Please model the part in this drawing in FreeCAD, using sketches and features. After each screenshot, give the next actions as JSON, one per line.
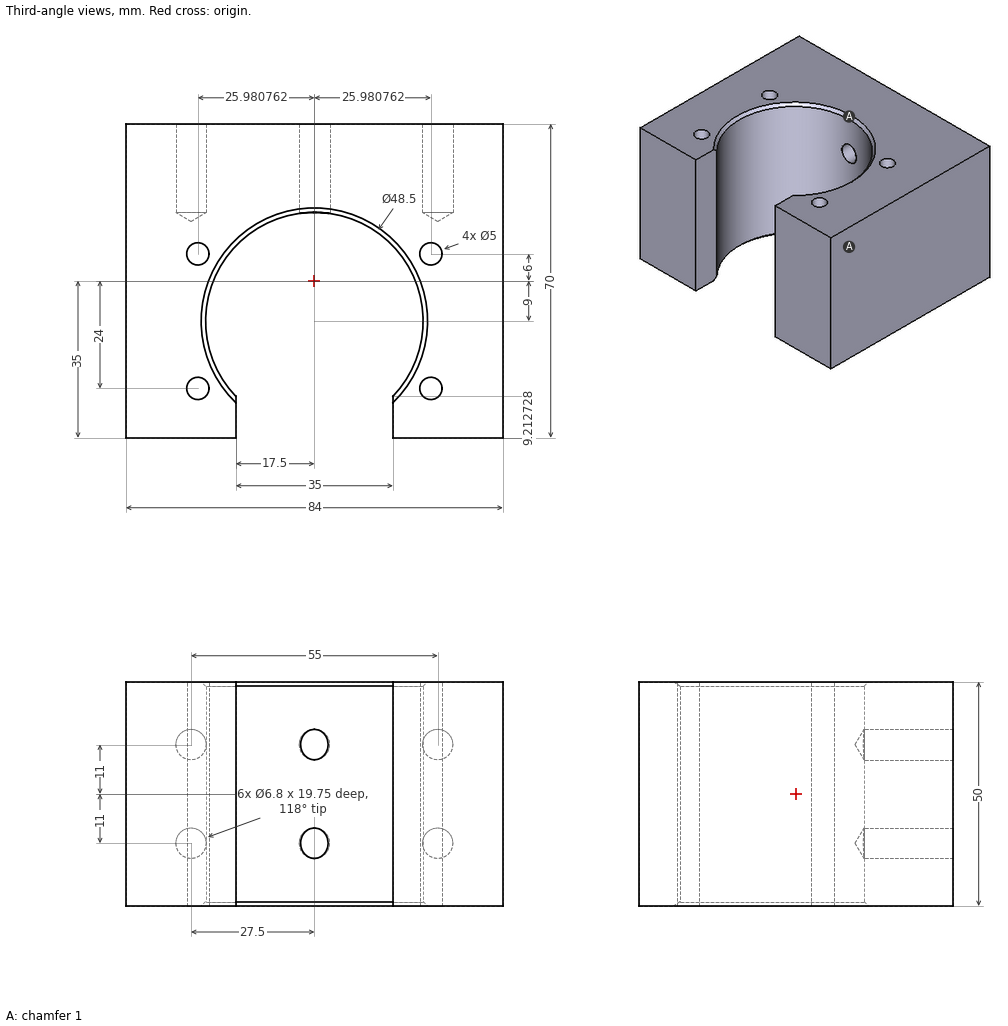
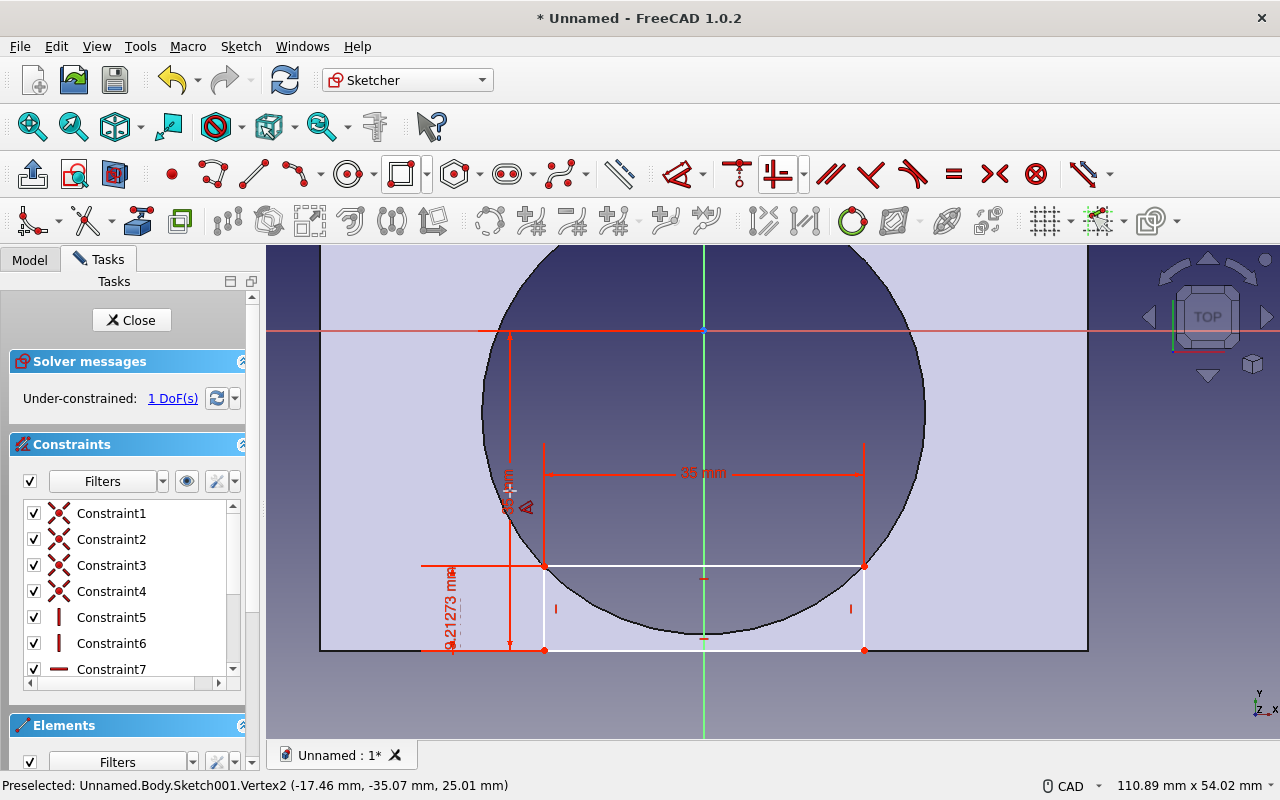
{"action": "left_click", "coordinate": [544, 566]}
{"action": "left_click", "coordinate": [624, 297]}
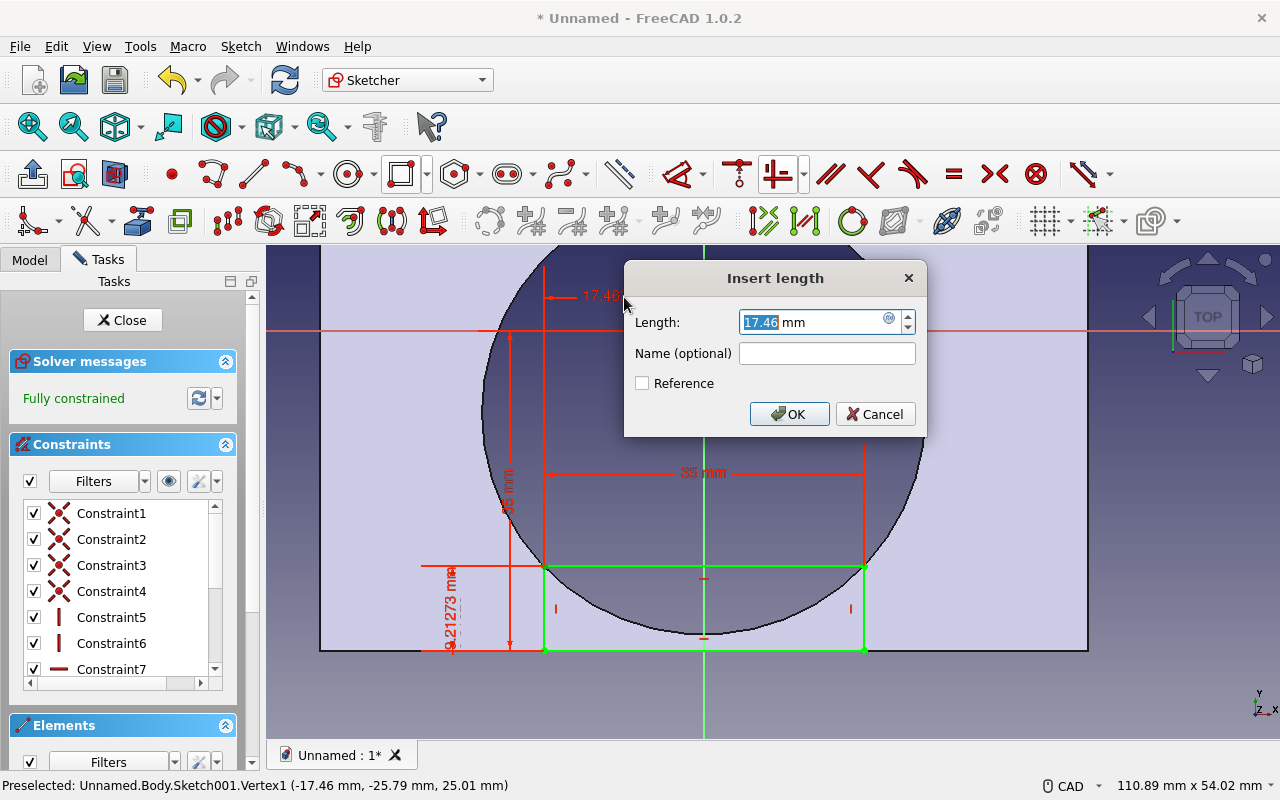
{"action": "type", "text": "17.5"}
{"action": "key", "text": "Return"}
{"action": "key", "text": "Escape"}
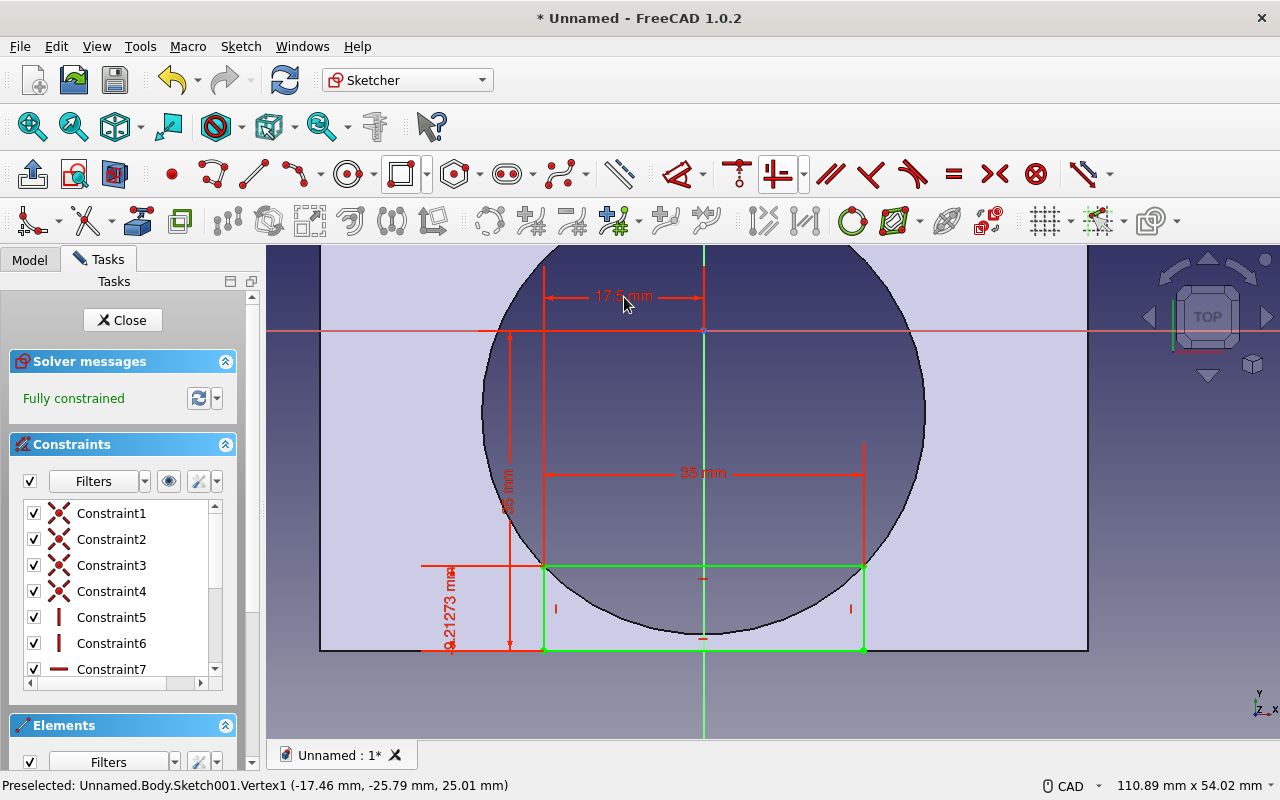
{"action": "left_click", "coordinate": [123, 320]}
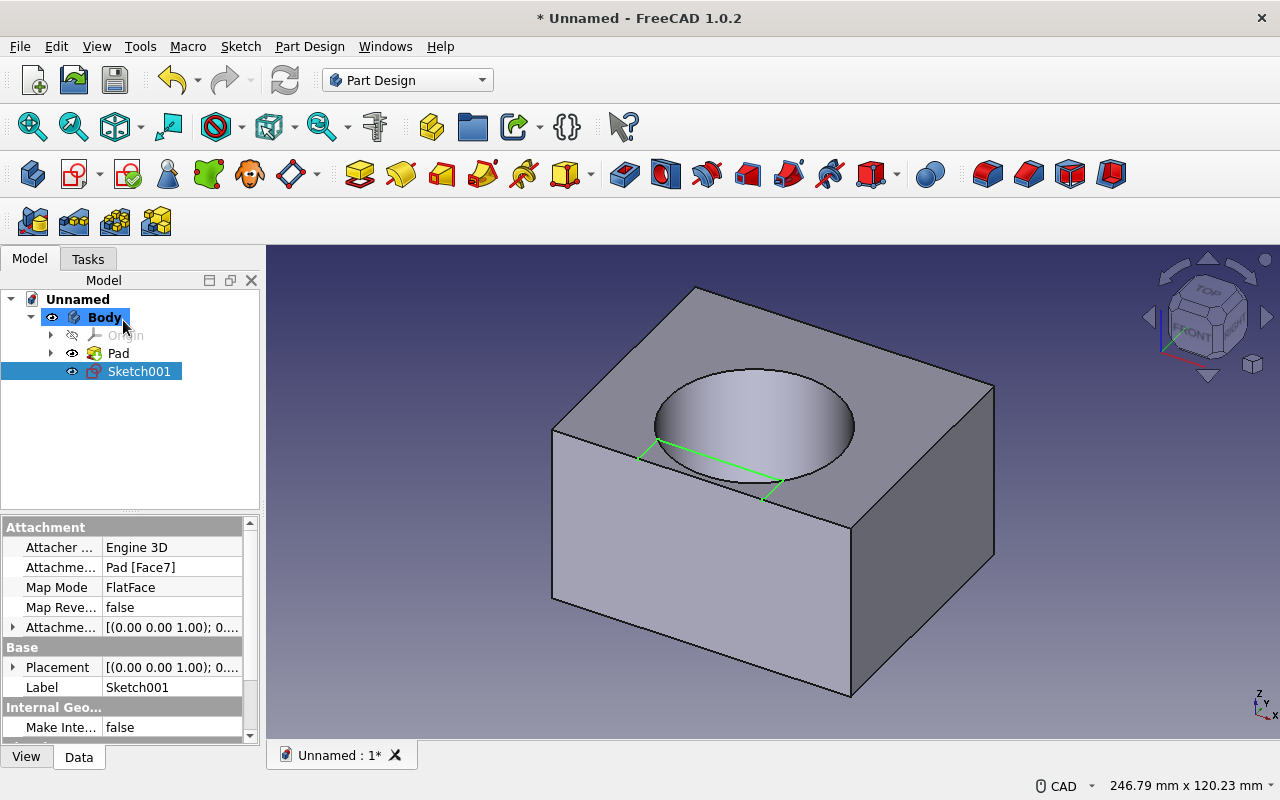
{"action": "left_click", "coordinate": [625, 174]}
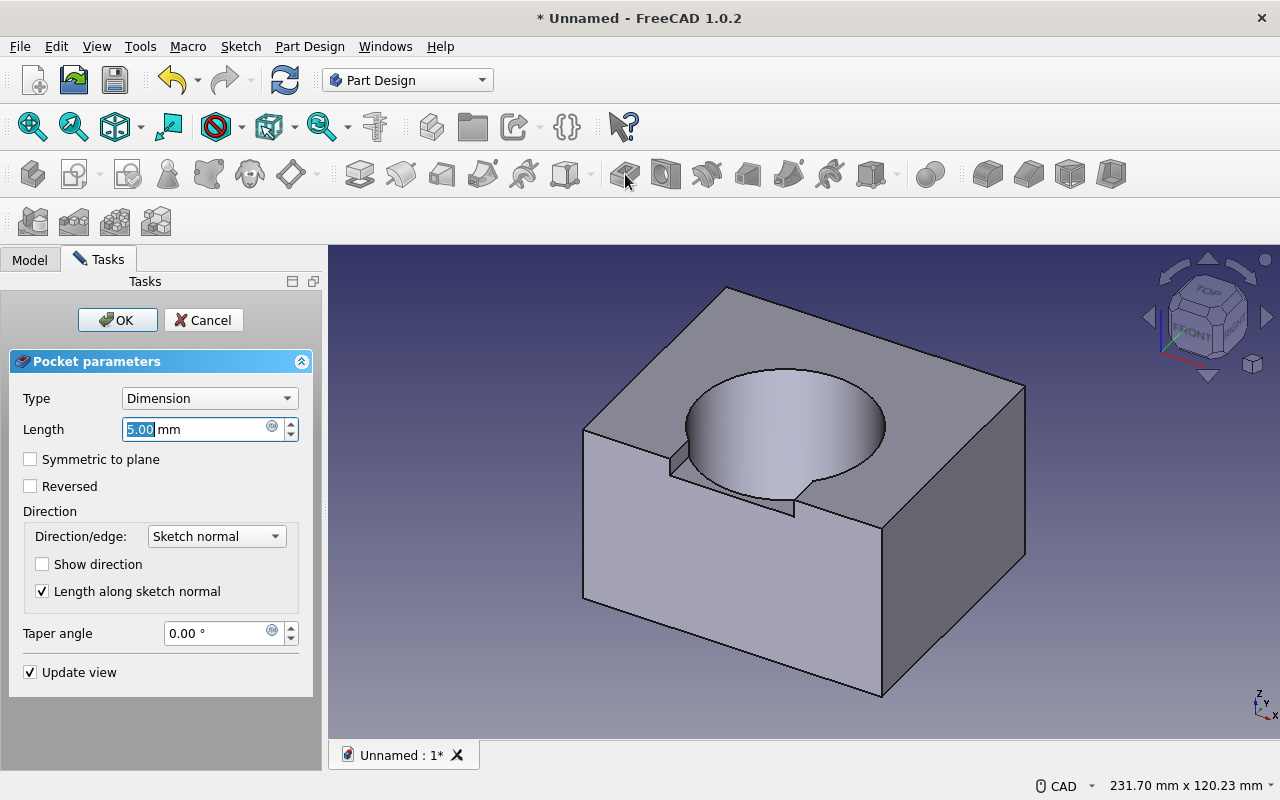
{"action": "left_click", "coordinate": [210, 398]}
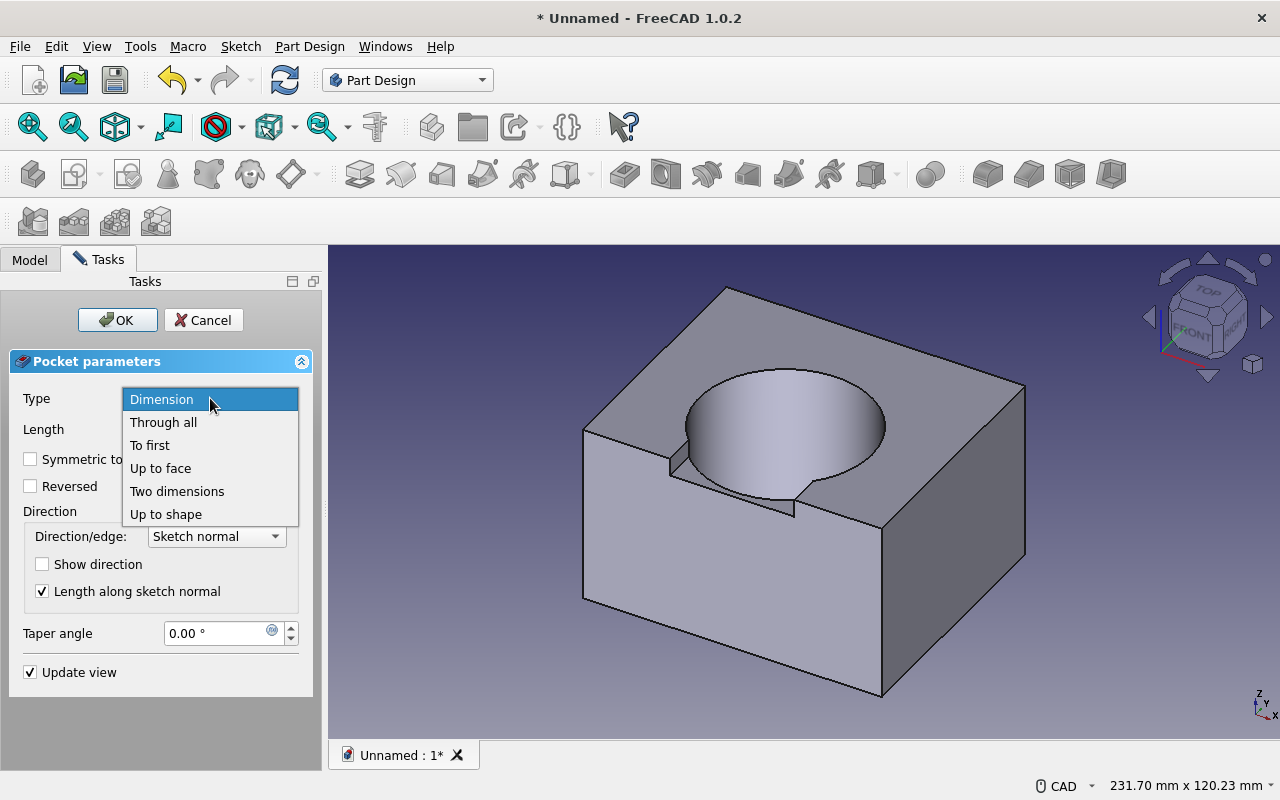
{"action": "left_click", "coordinate": [208, 422]}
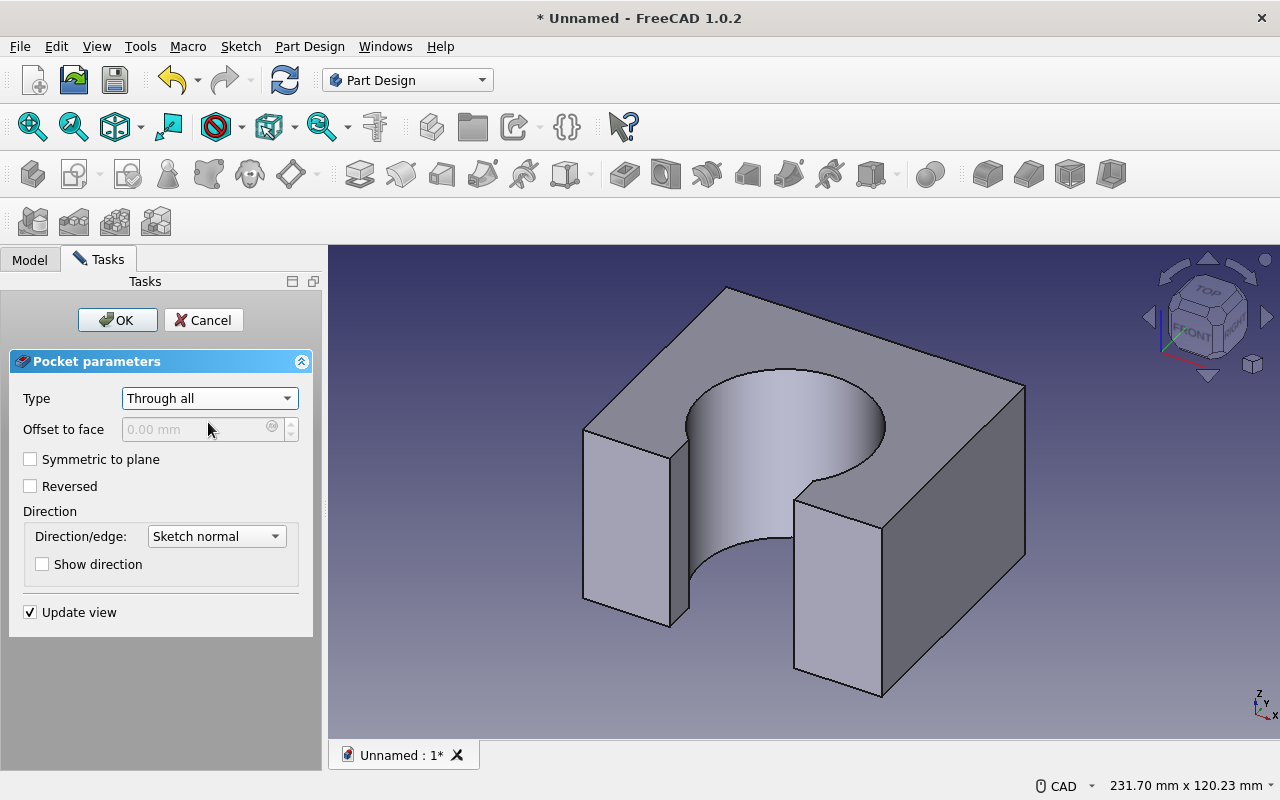
{"action": "left_click", "coordinate": [118, 320]}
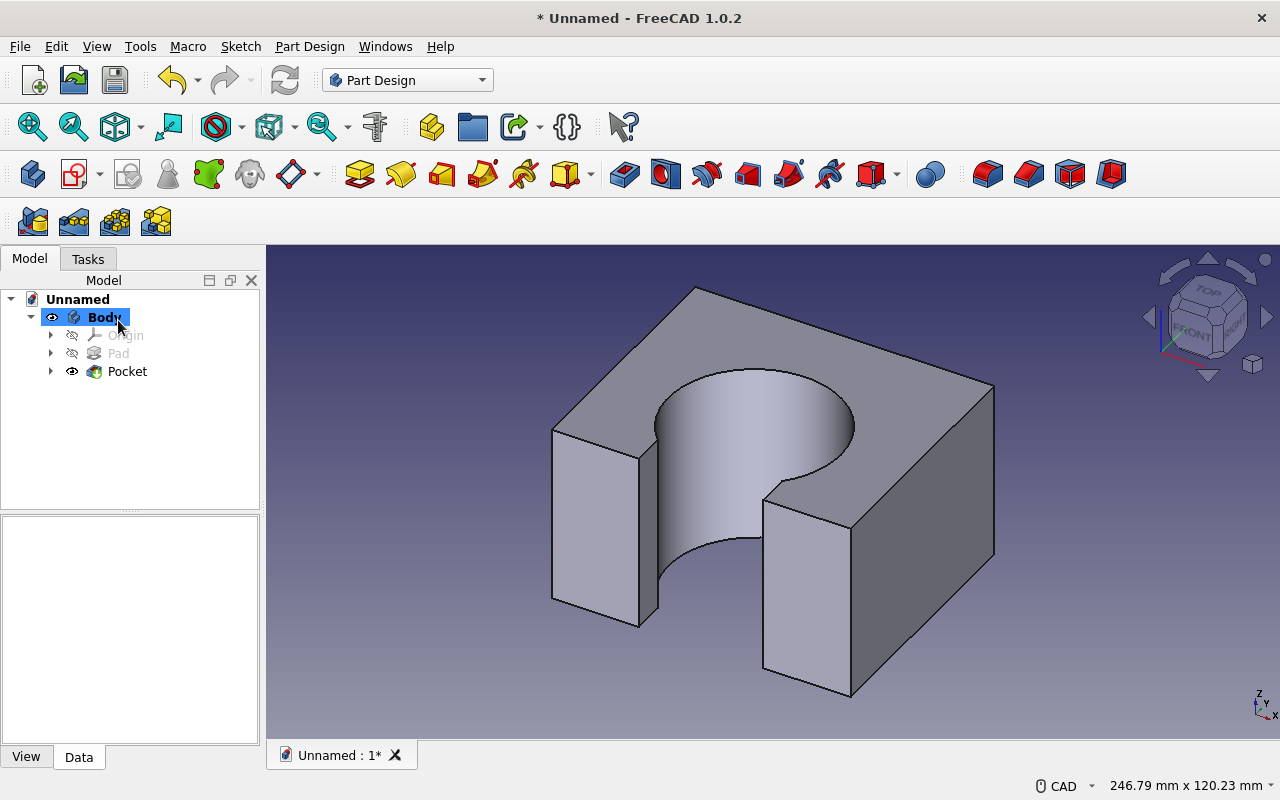
{"action": "key", "text": "5"}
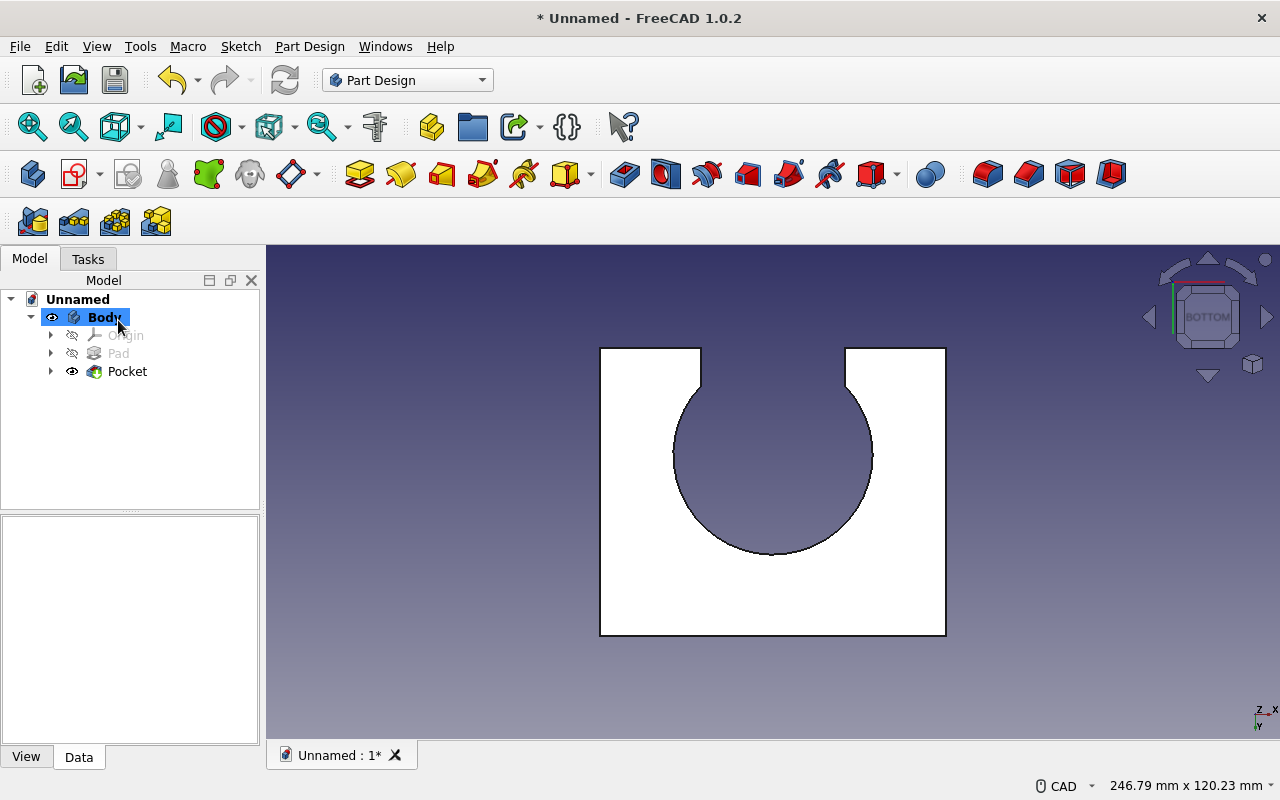
{"action": "left_click", "coordinate": [872, 573]}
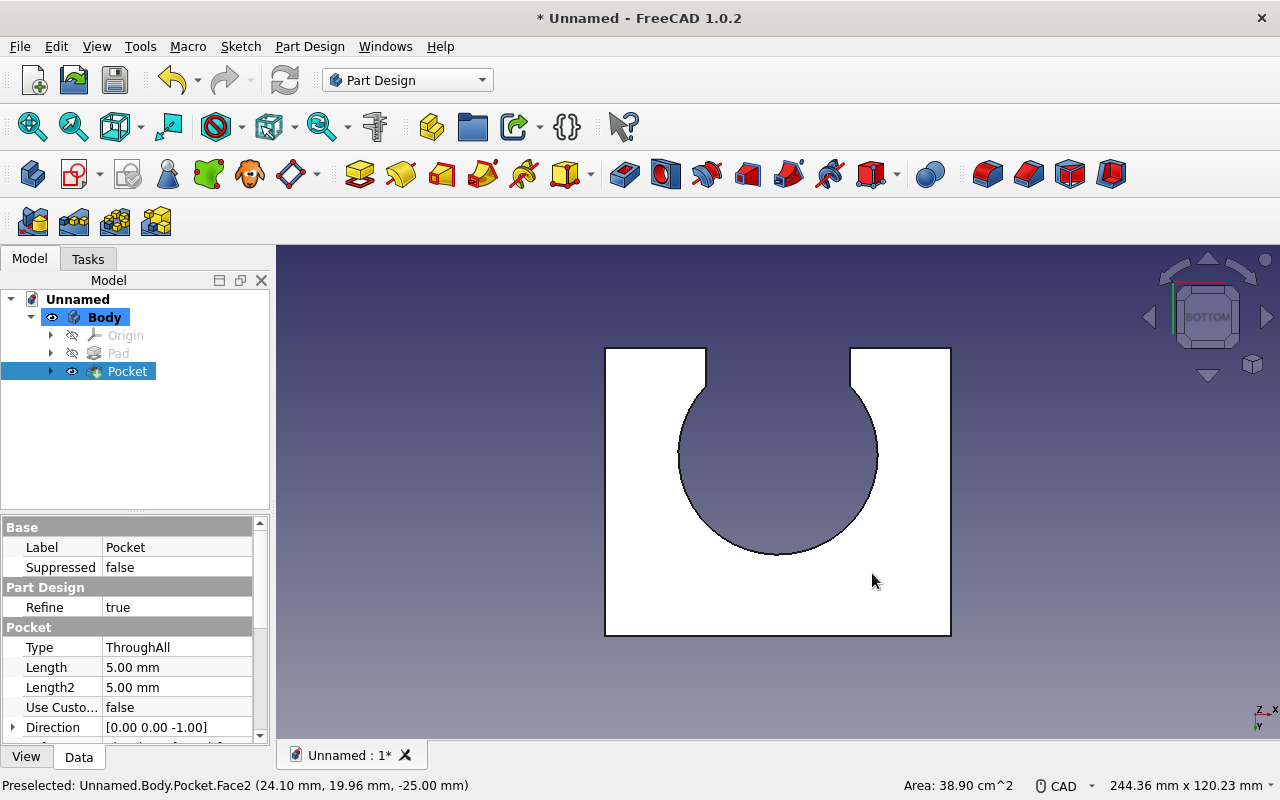
{"action": "left_click", "coordinate": [74, 174]}